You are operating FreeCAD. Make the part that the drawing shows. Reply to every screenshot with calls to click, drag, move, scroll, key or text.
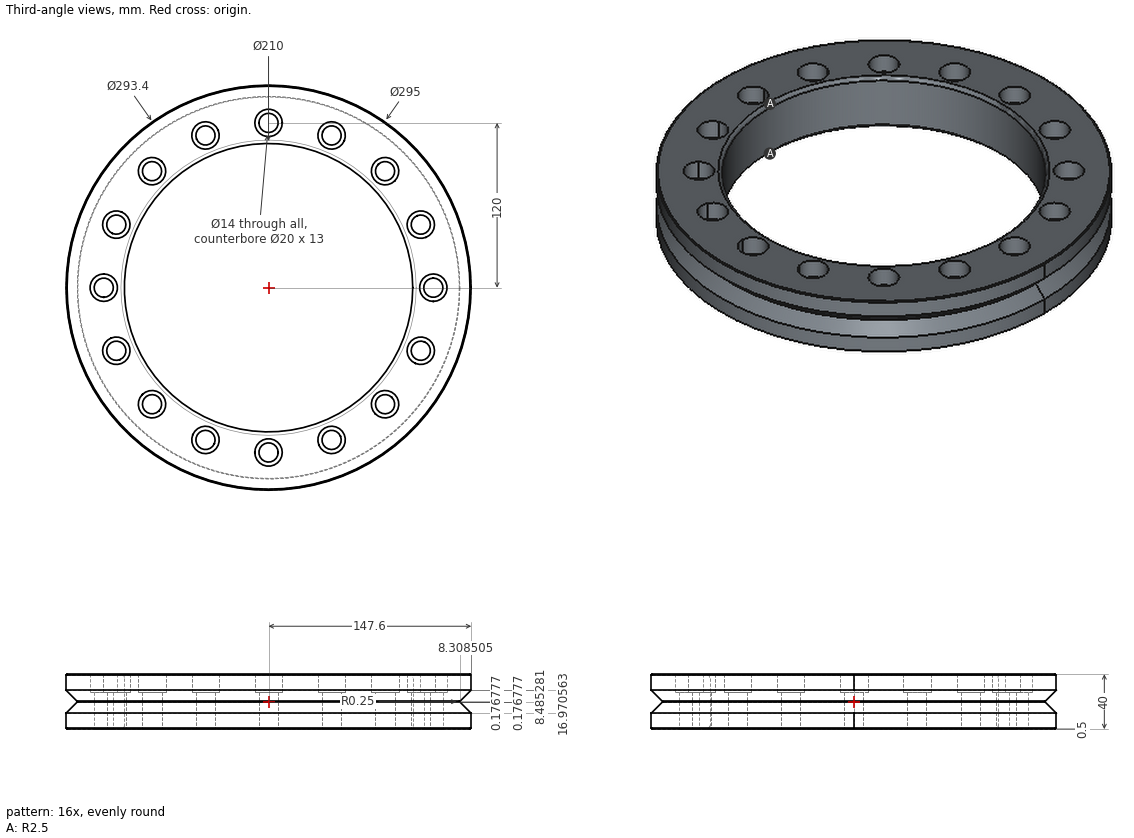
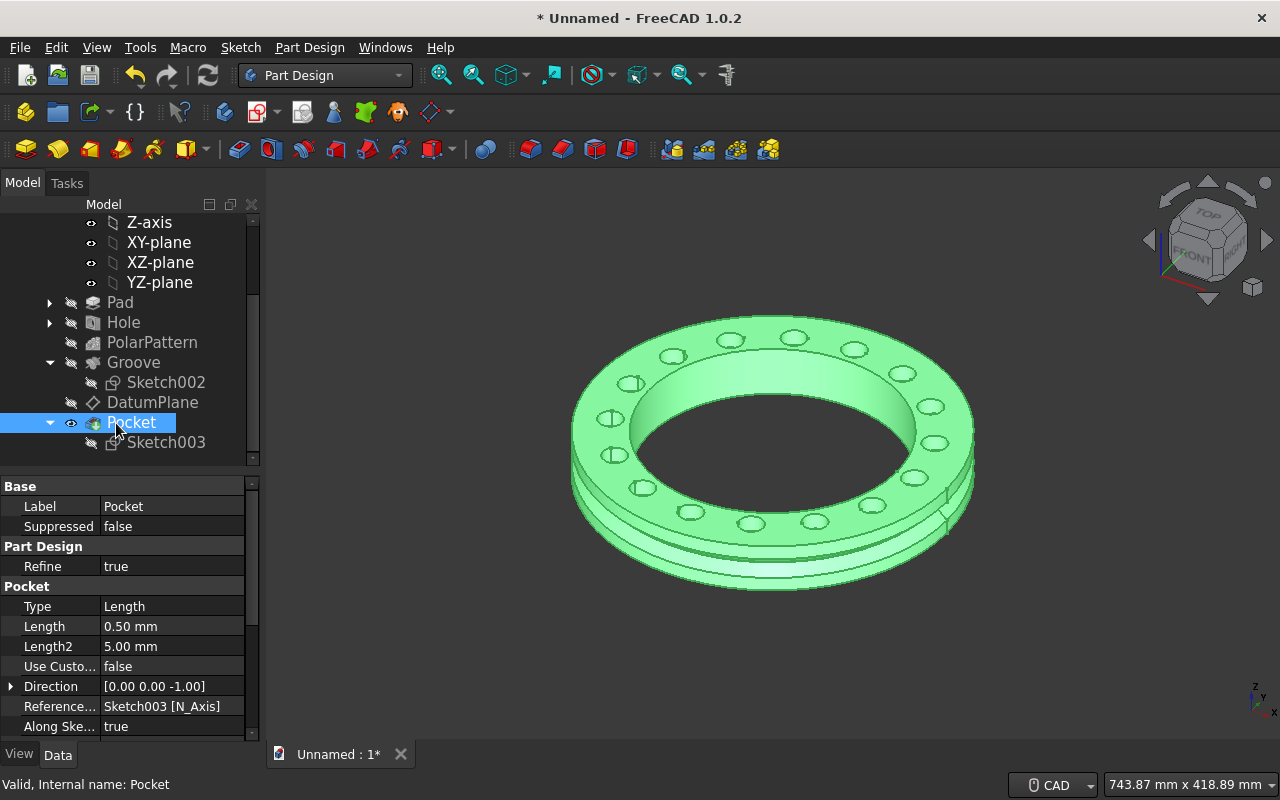
click(672, 150)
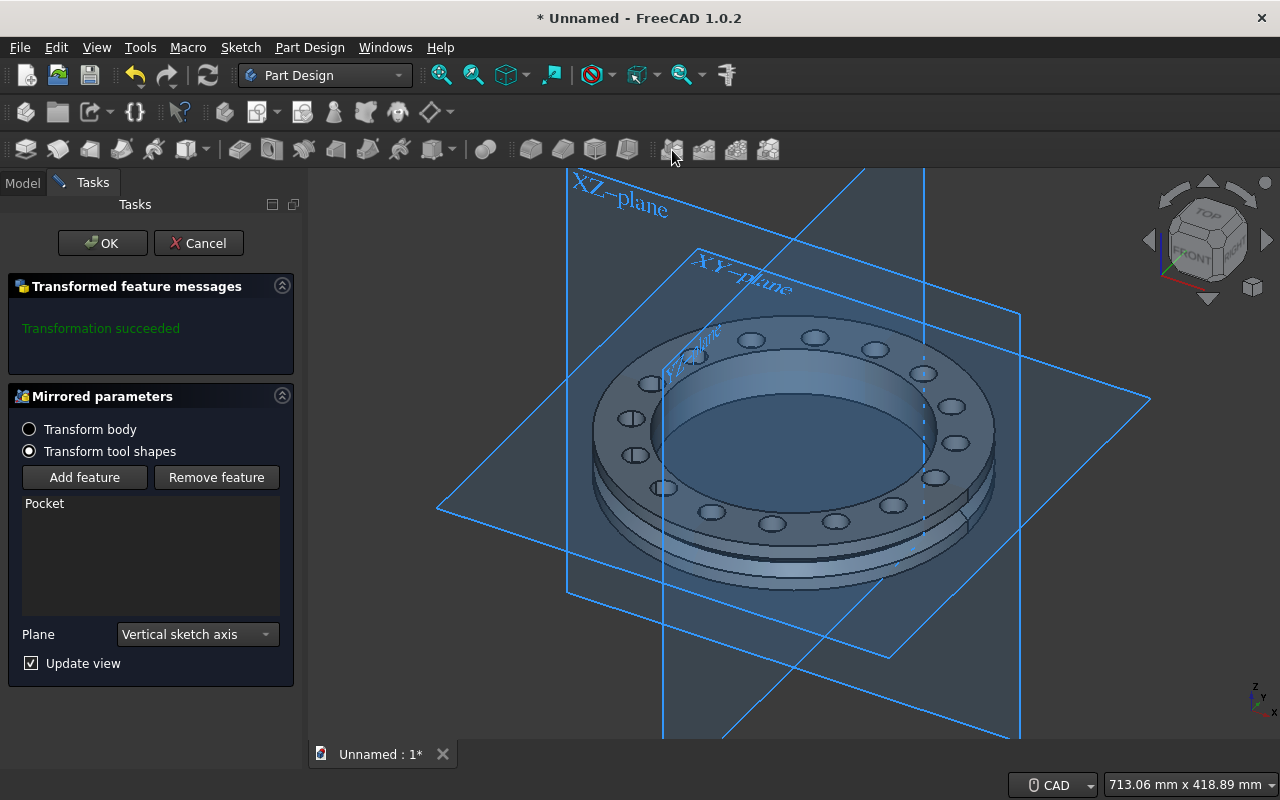
click(198, 634)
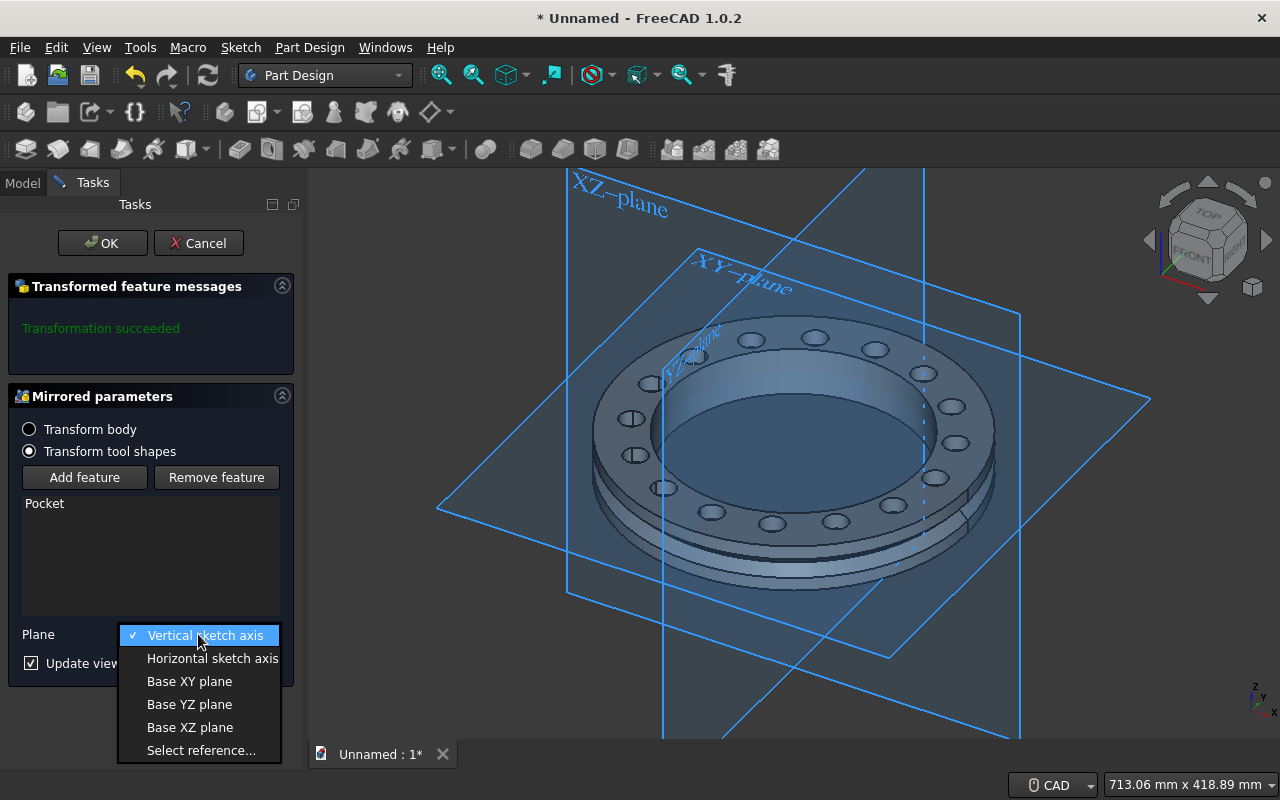
click(198, 682)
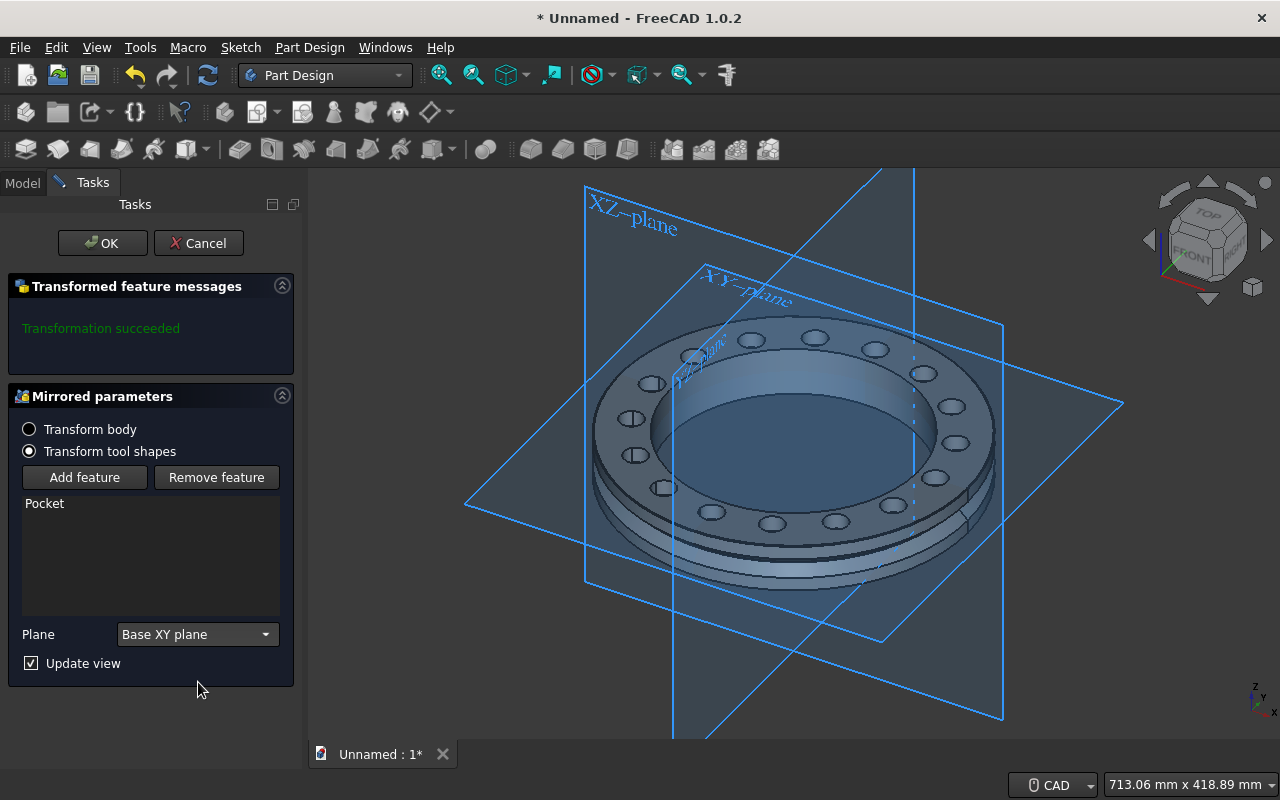
click(103, 243)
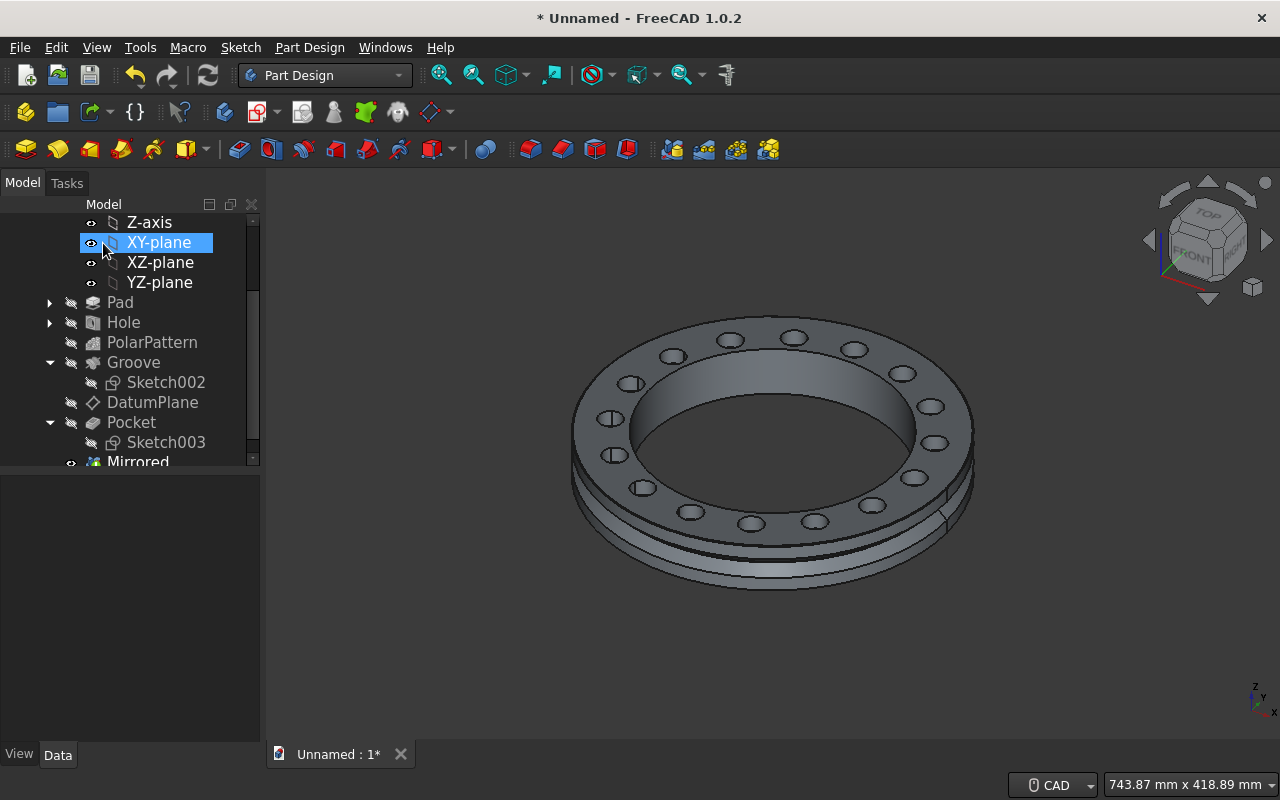
click(649, 389)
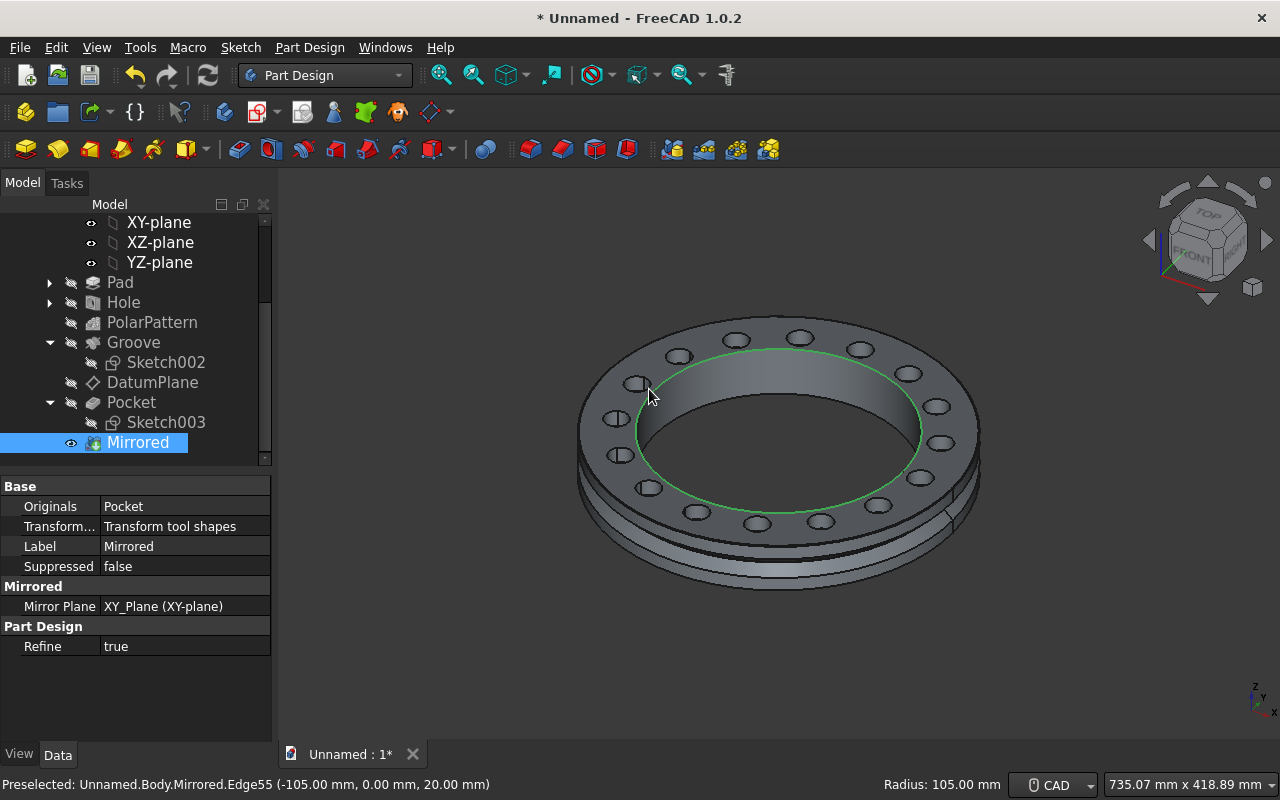
key(0)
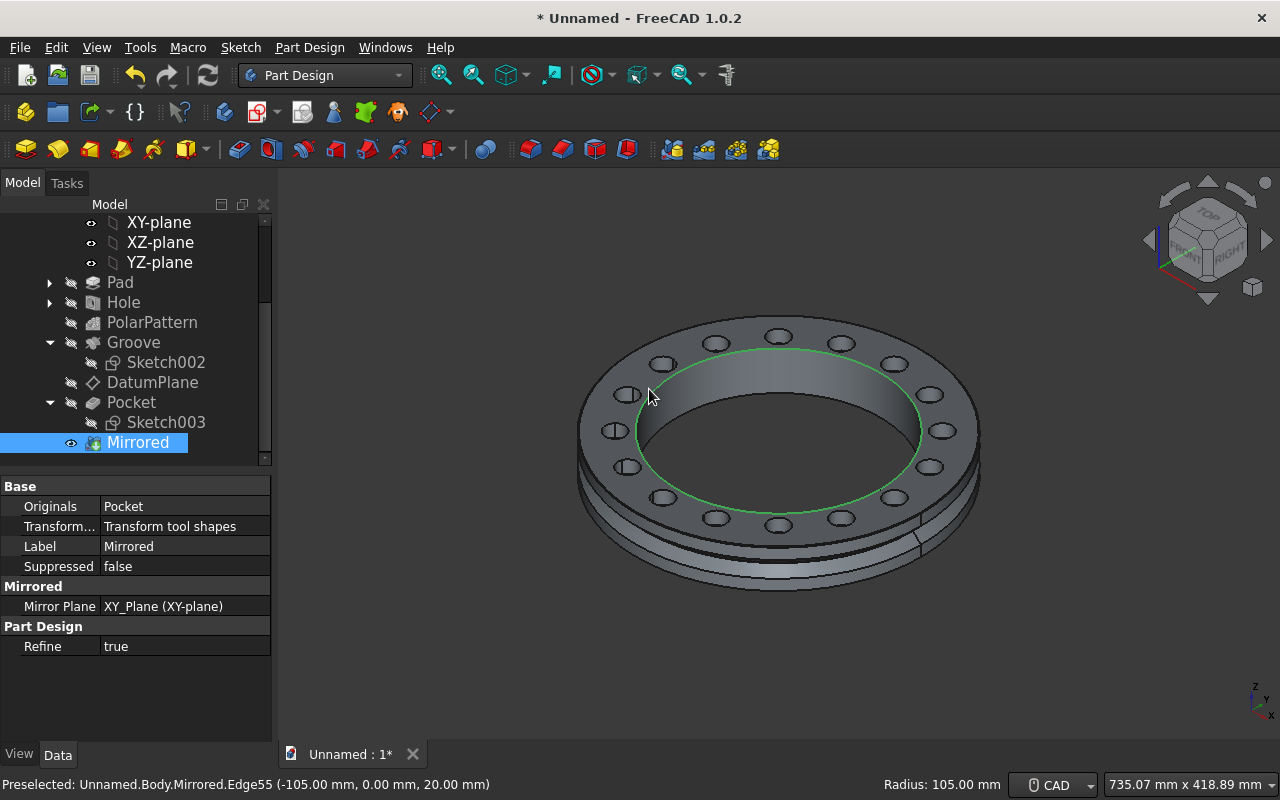
key(2)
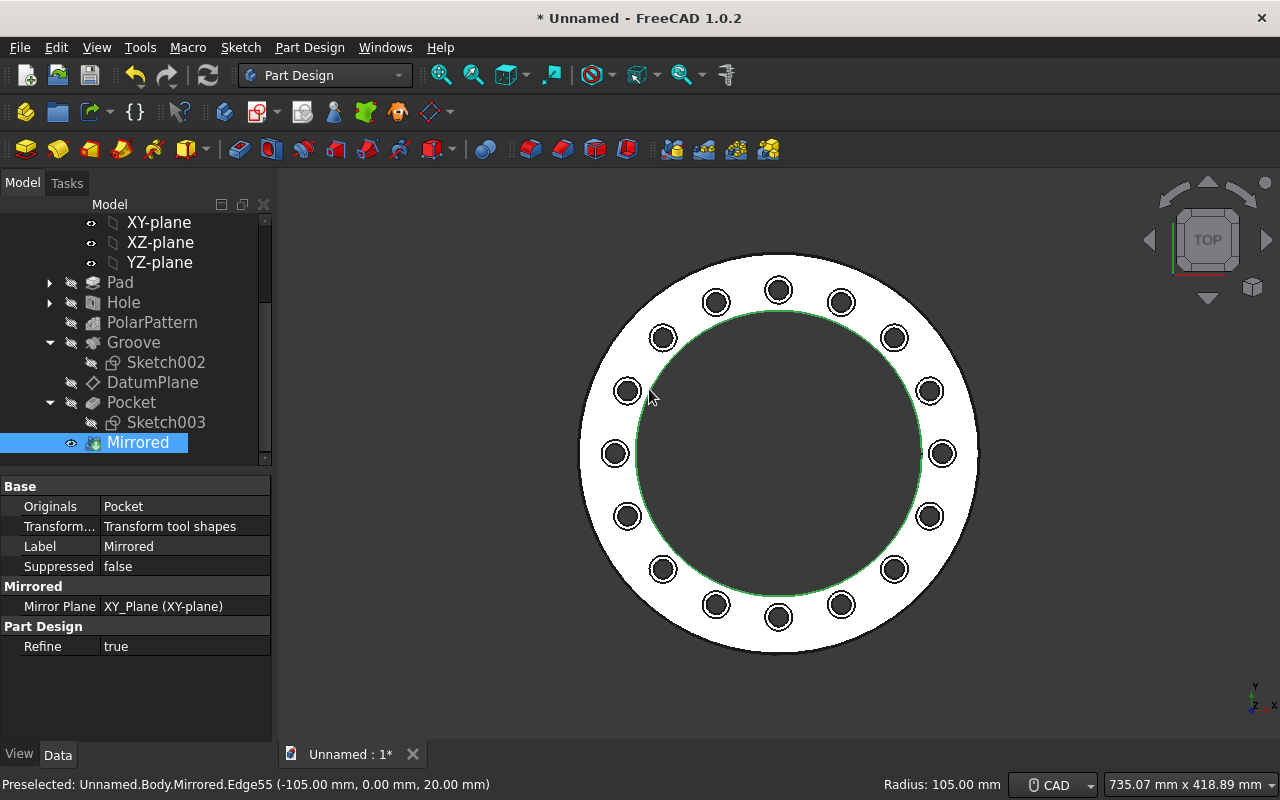
key(1)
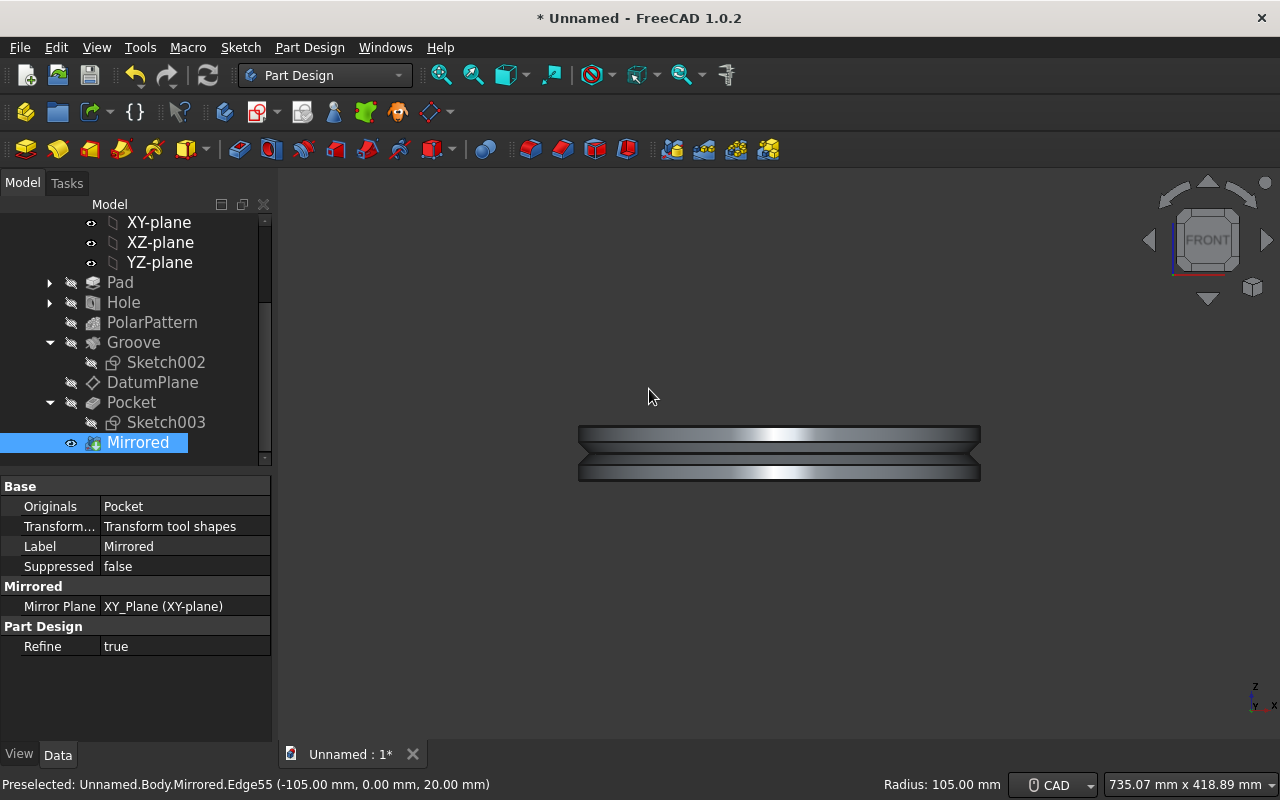
click(442, 76)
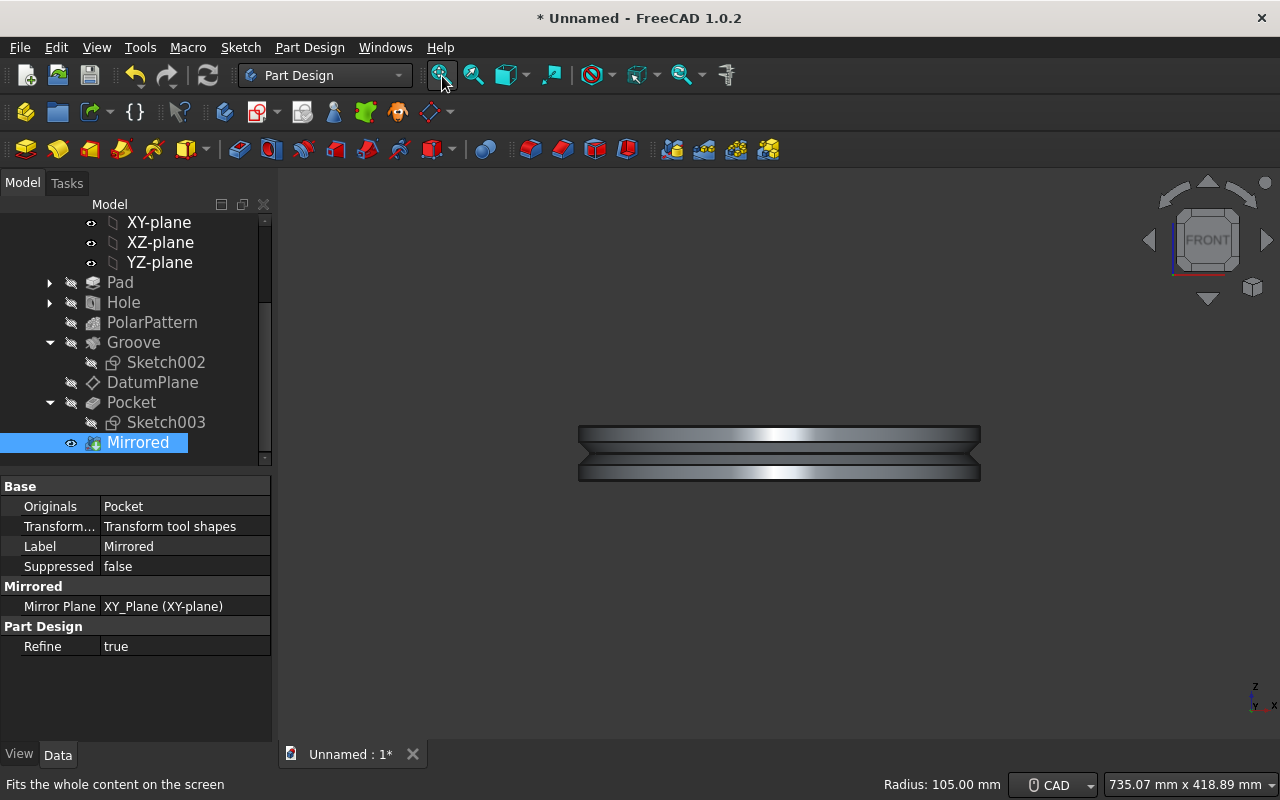
key(3)